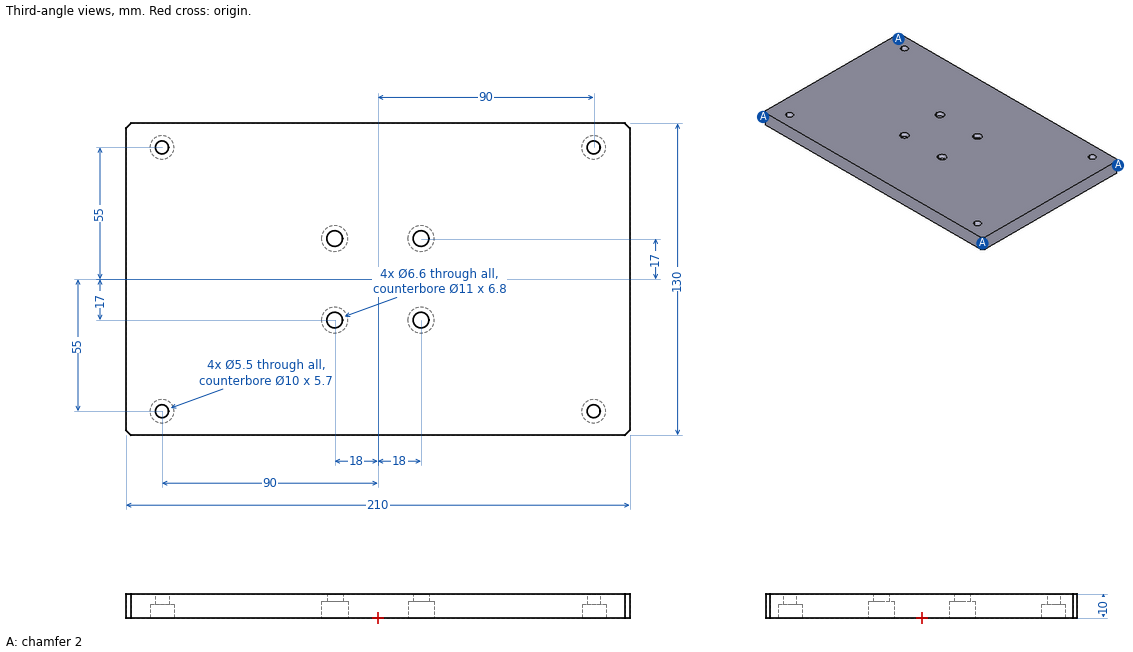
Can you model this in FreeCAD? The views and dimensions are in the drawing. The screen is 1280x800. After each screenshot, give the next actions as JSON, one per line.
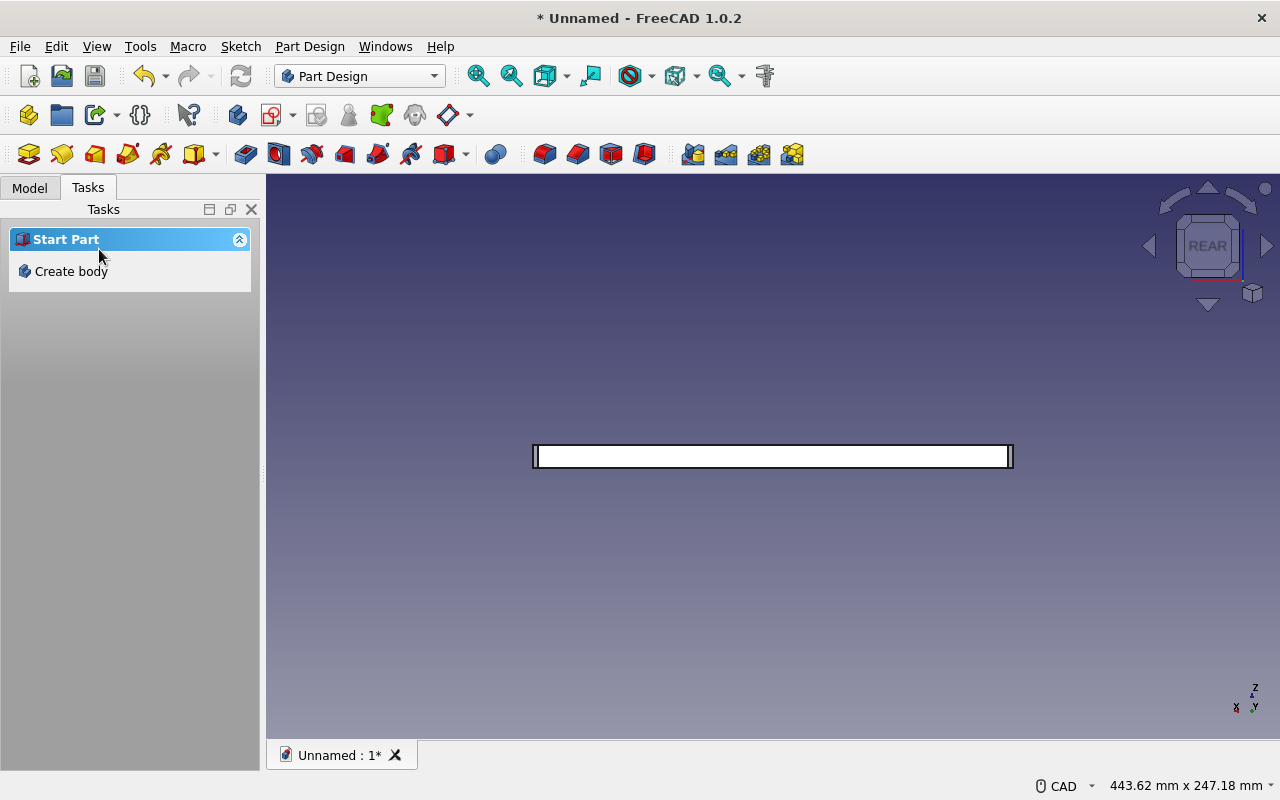
{"action": "key", "text": "0"}